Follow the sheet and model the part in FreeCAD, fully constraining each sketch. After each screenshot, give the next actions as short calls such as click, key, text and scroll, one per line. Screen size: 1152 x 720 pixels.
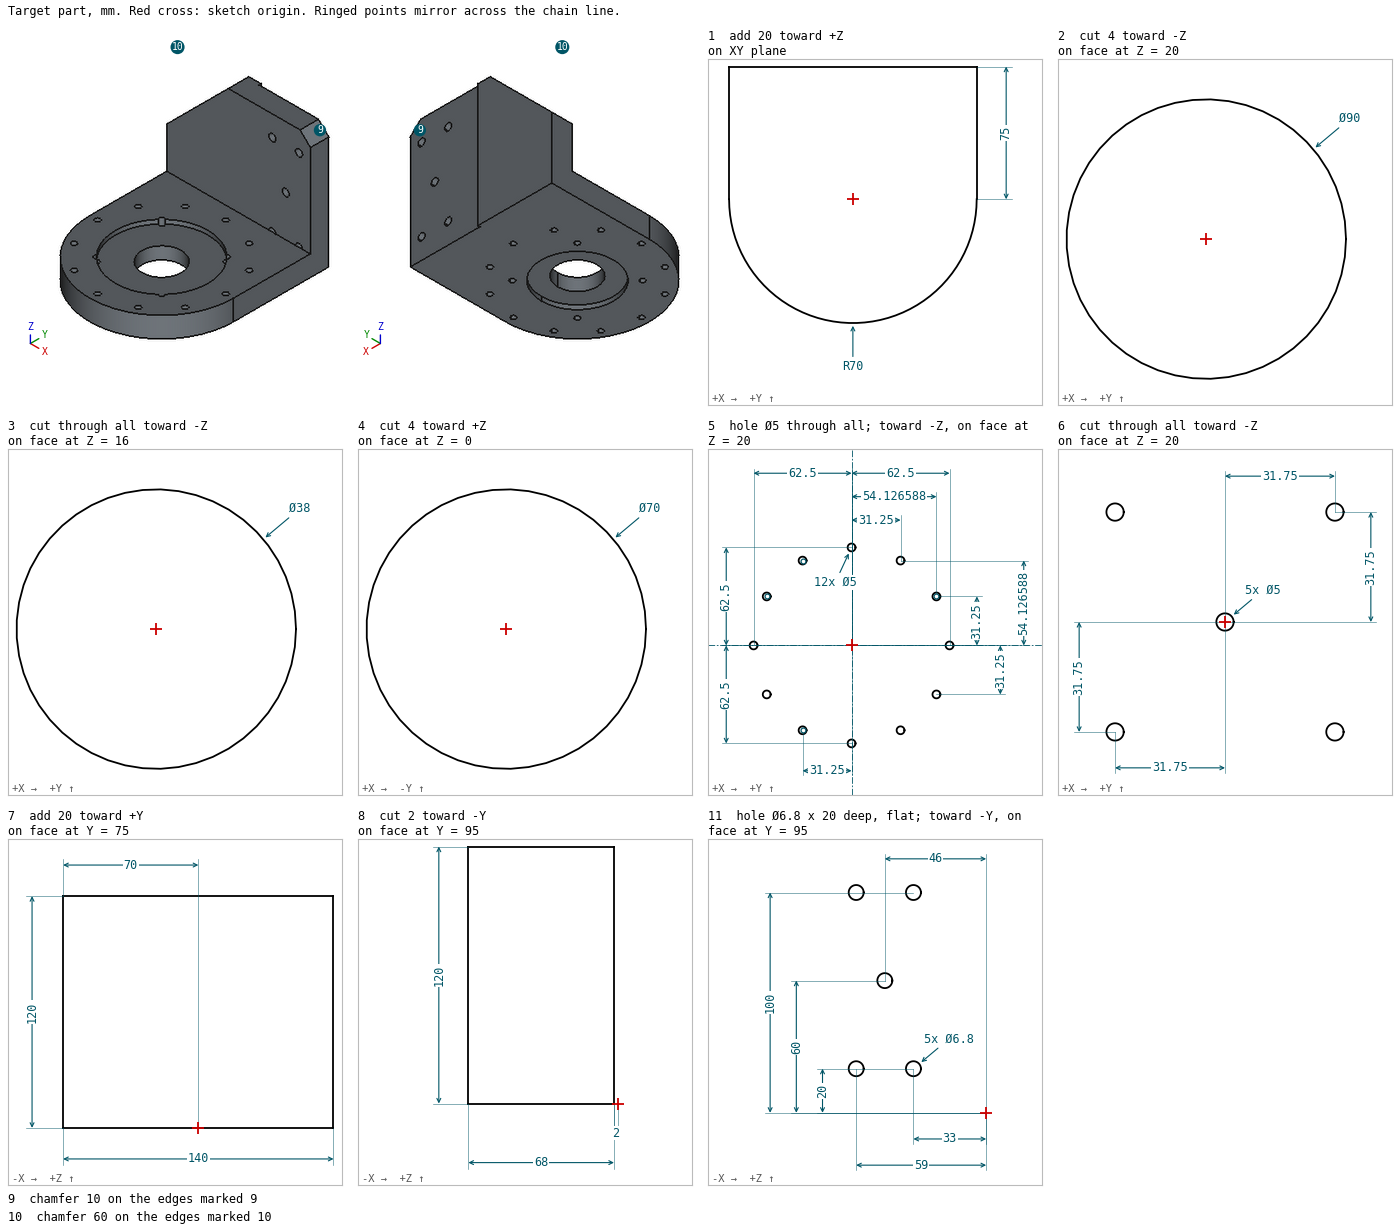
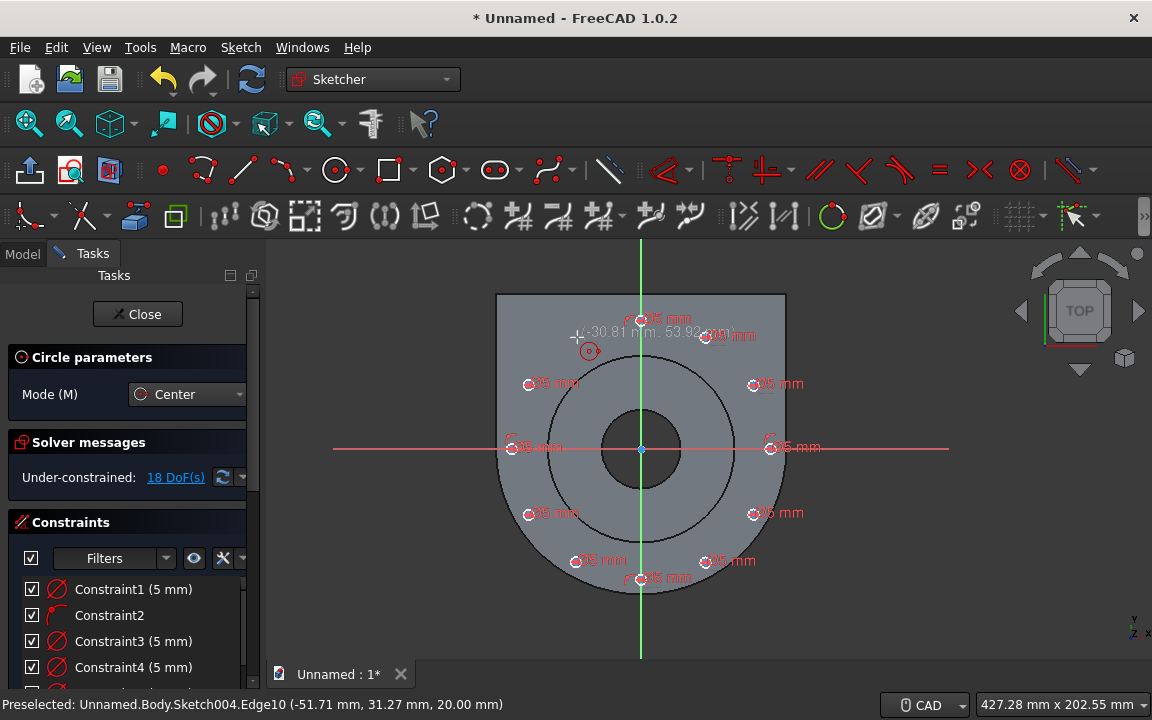
click(576, 337)
move(580, 333)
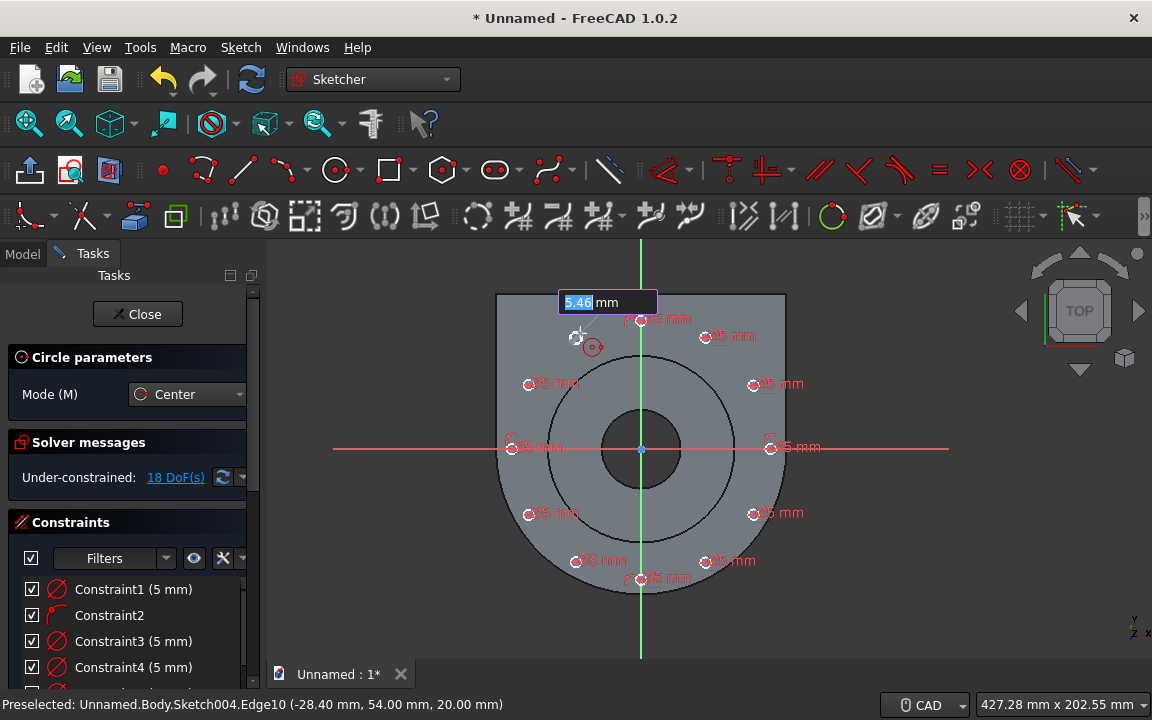
text(5)
key(Return)
key(Escape)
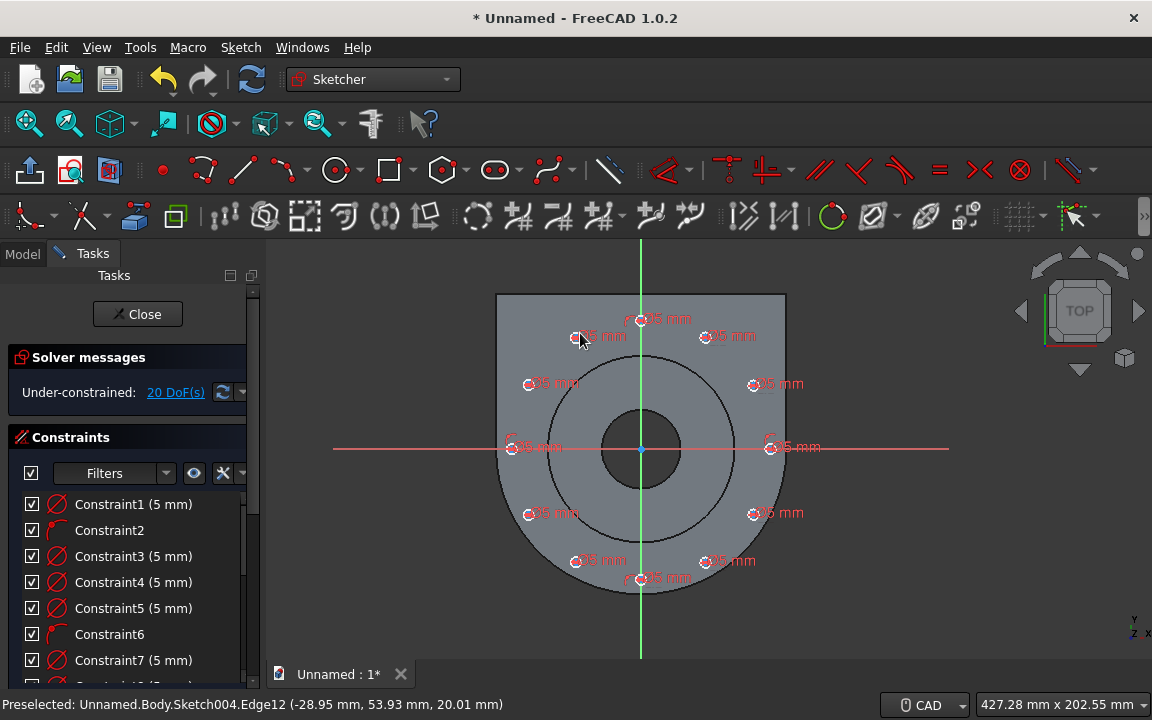
click(754, 386)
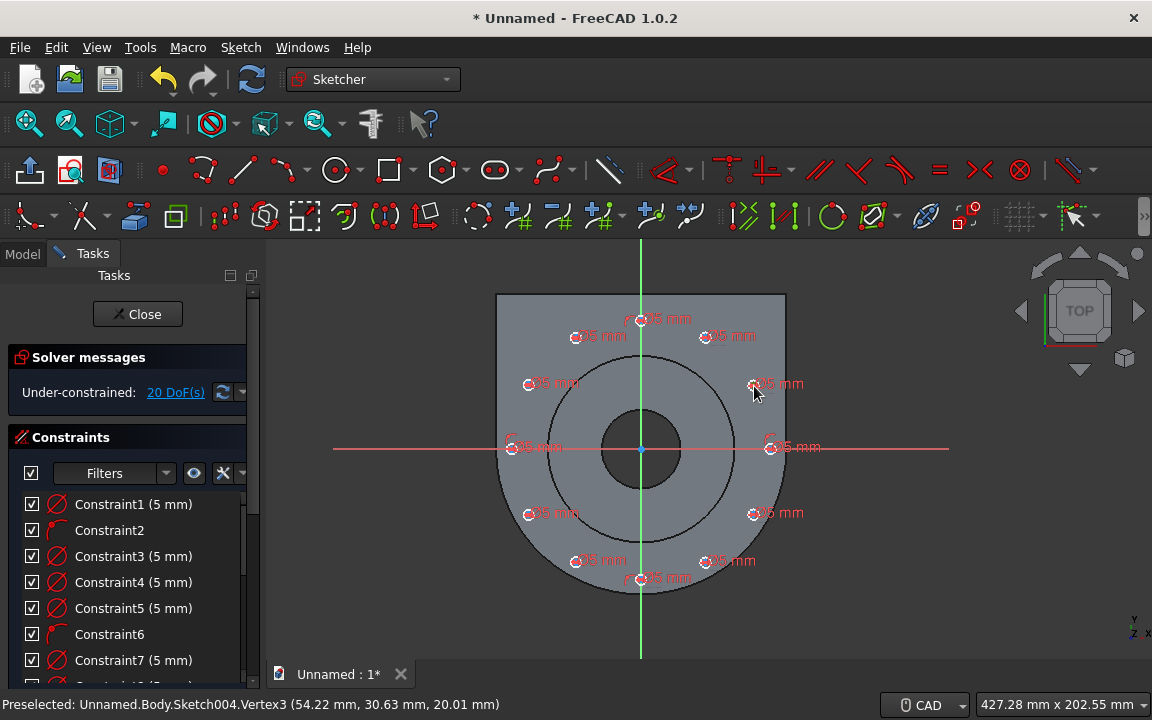
click(754, 515)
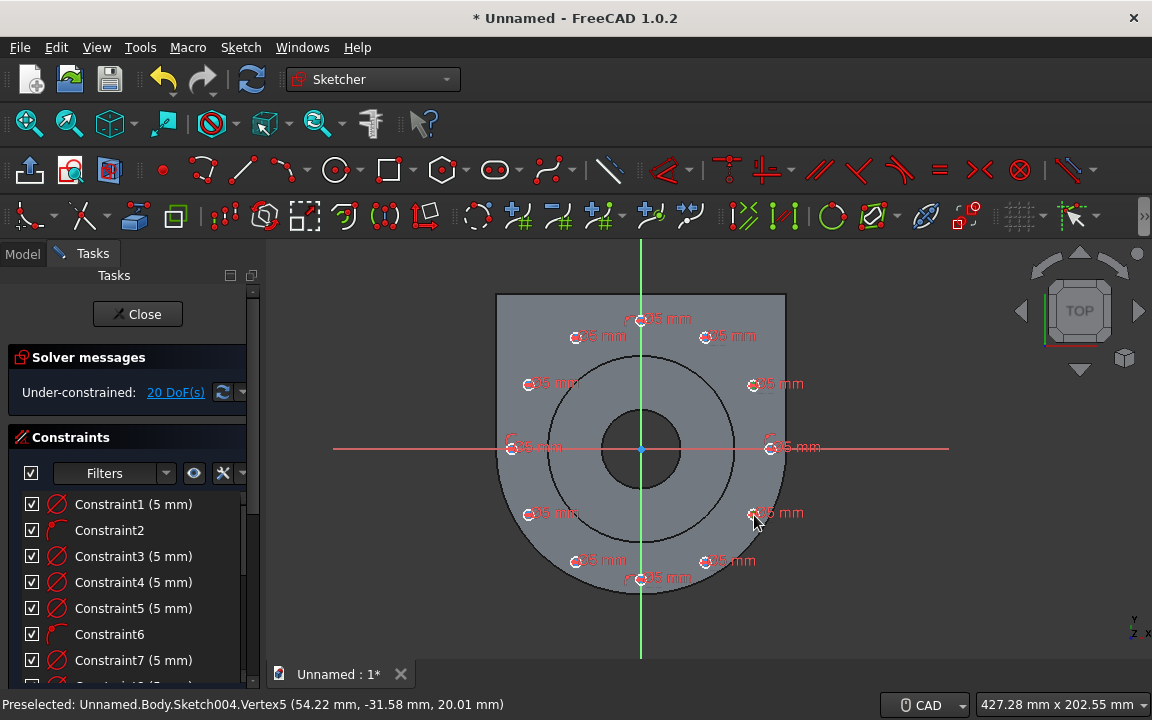
key(v)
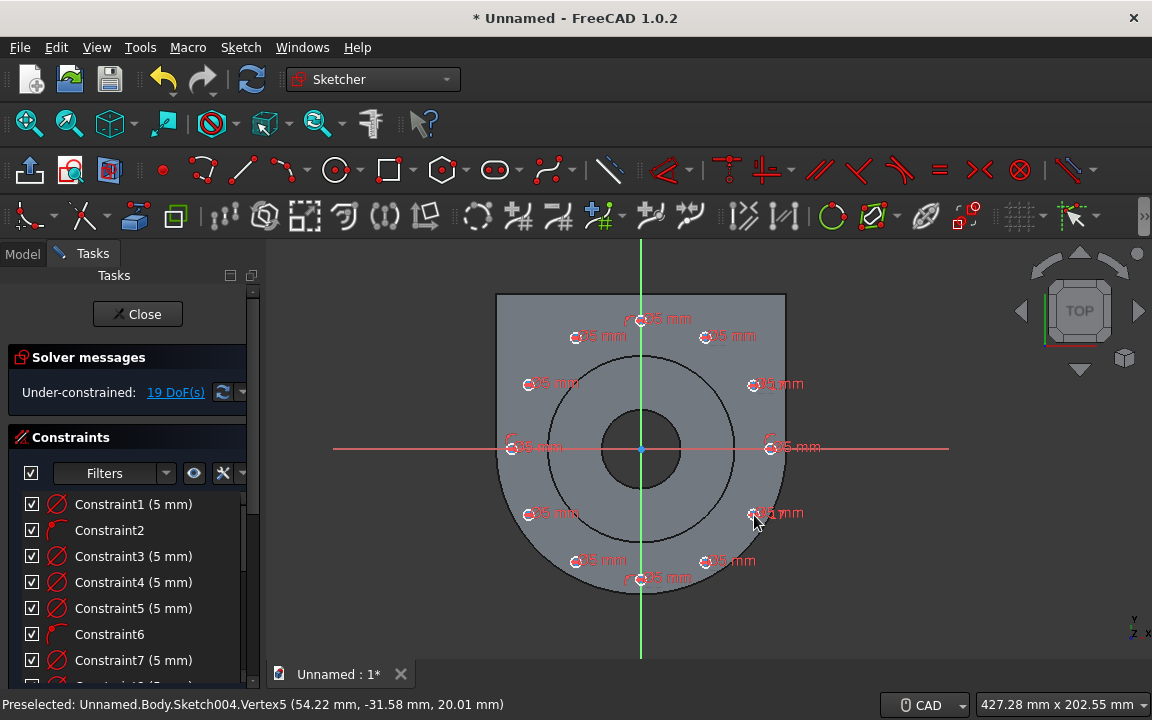
click(706, 338)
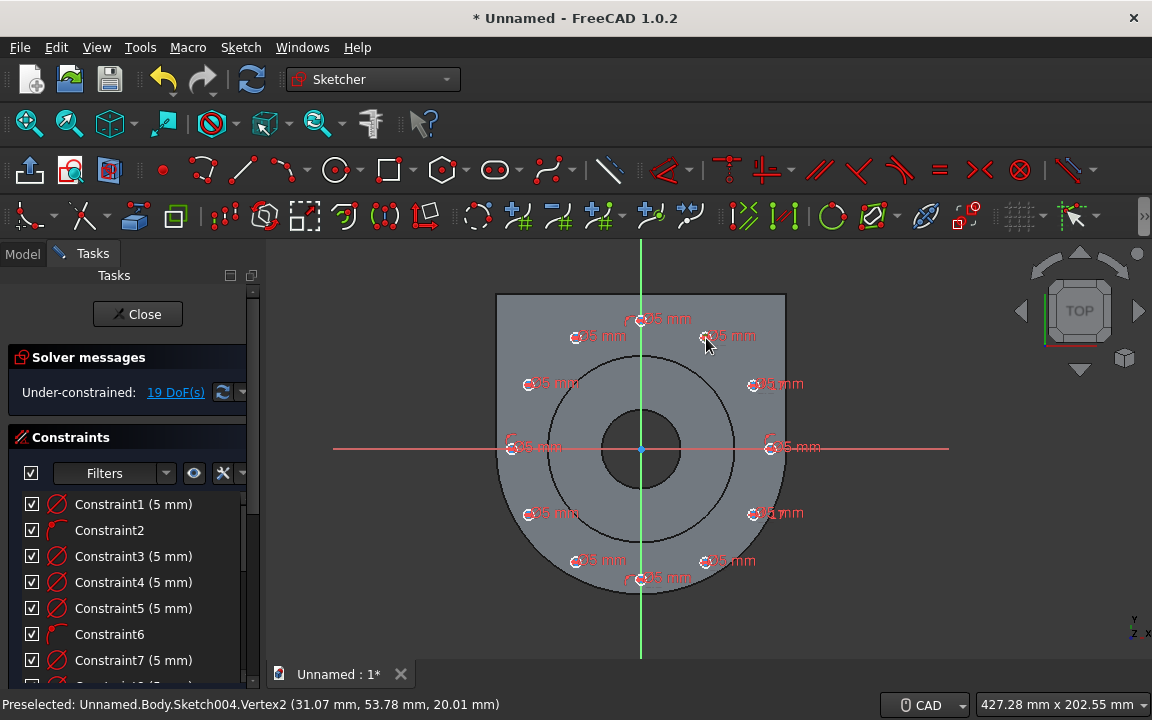
click(706, 563)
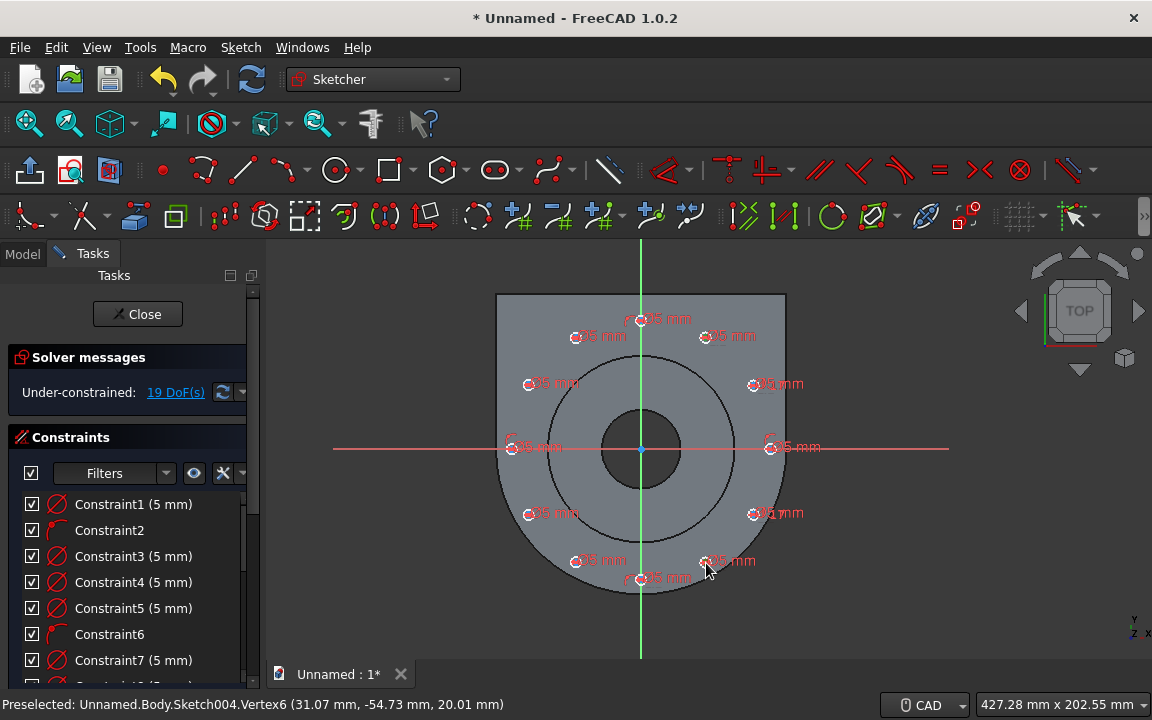
key(v)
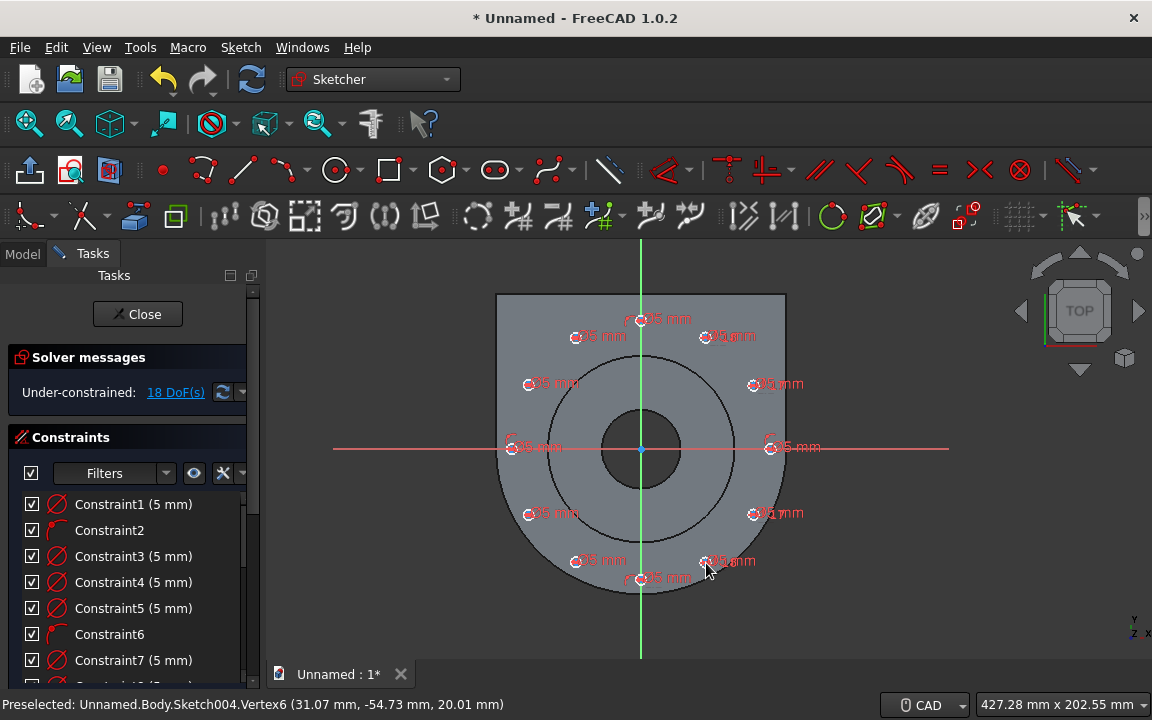
click(706, 563)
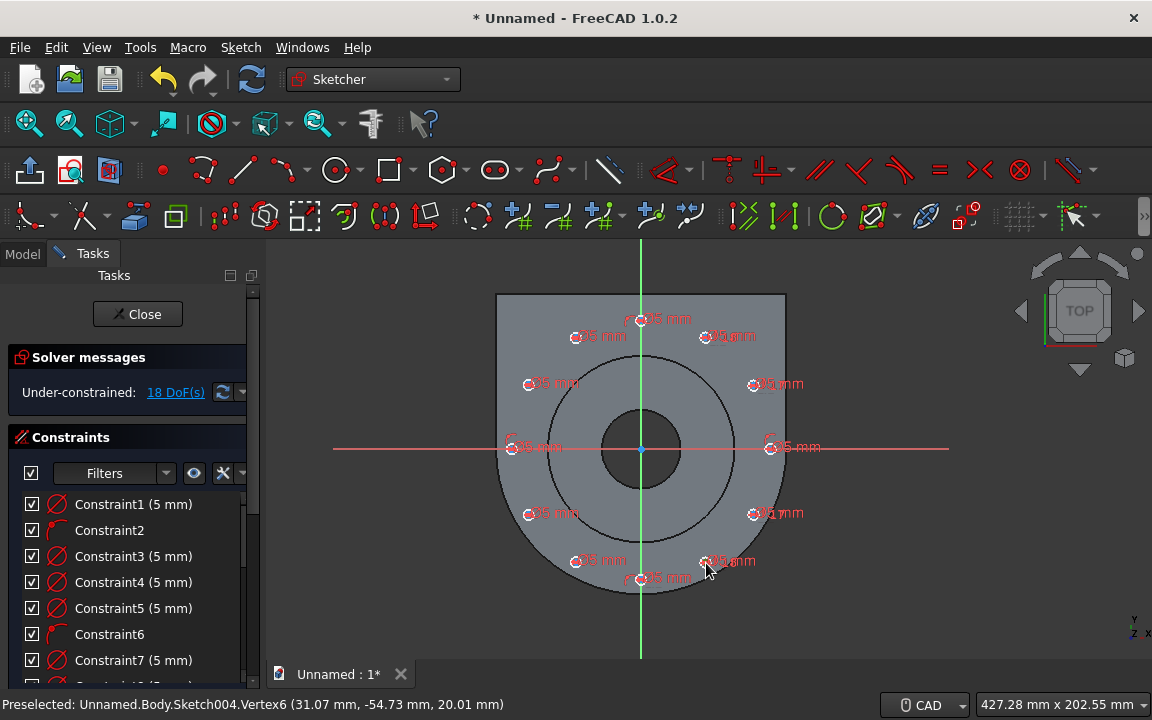
click(576, 562)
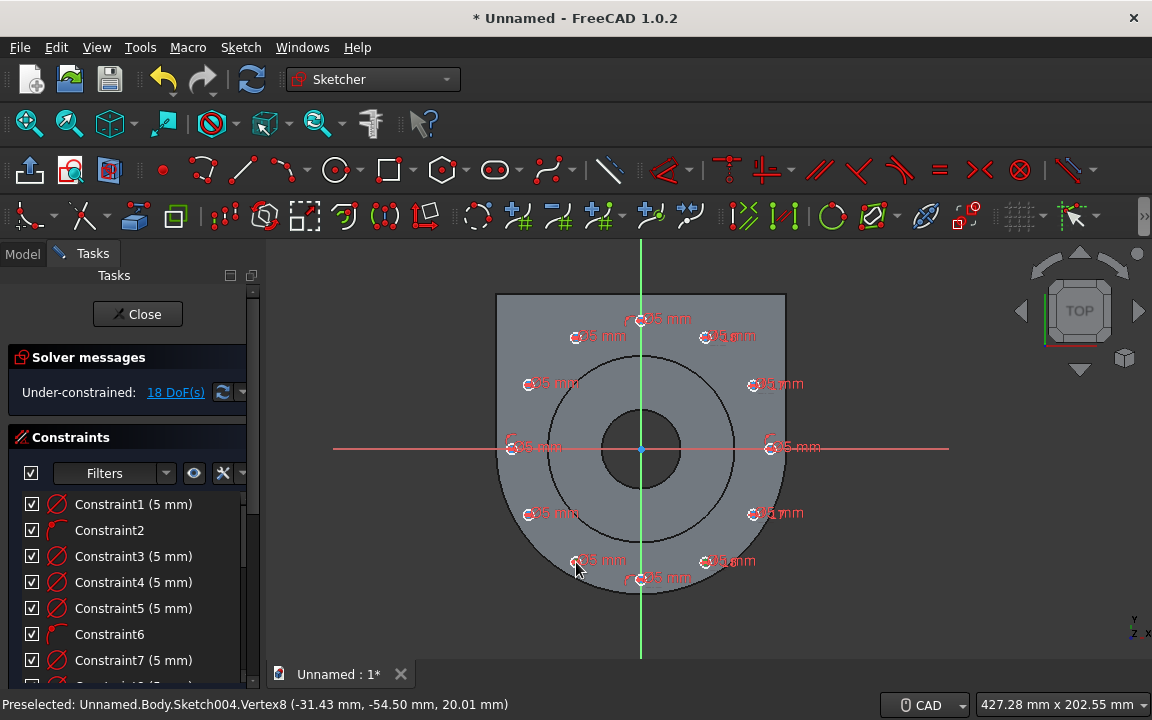
key(h)